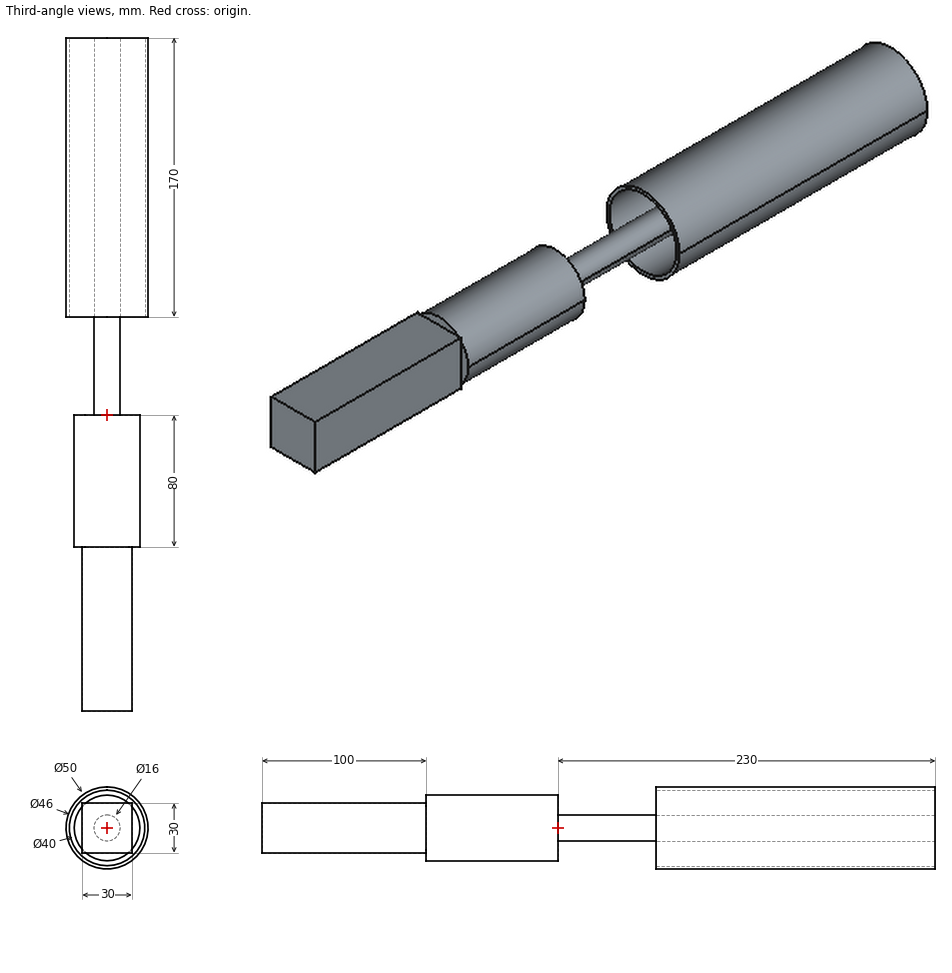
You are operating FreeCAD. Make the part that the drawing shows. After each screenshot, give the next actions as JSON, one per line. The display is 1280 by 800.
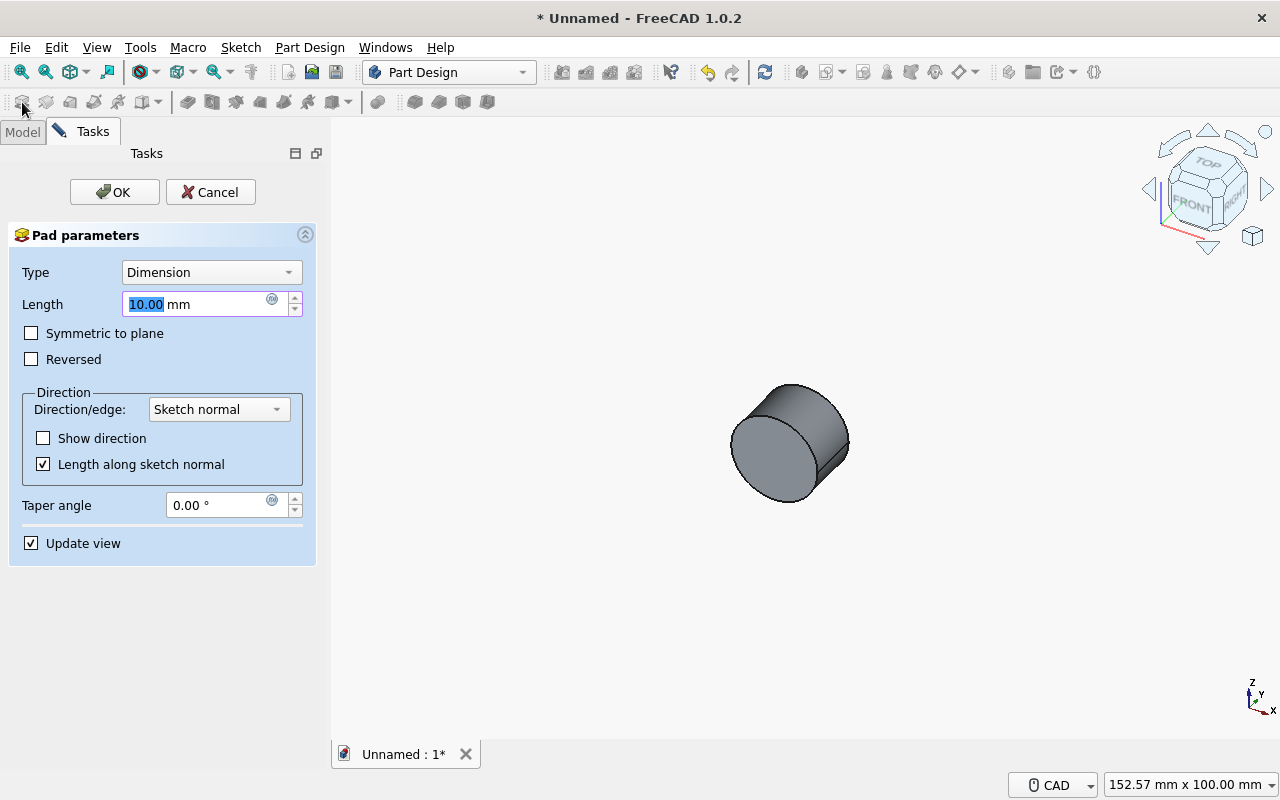
{"action": "type", "text": "230"}
{"action": "key", "text": "Tab"}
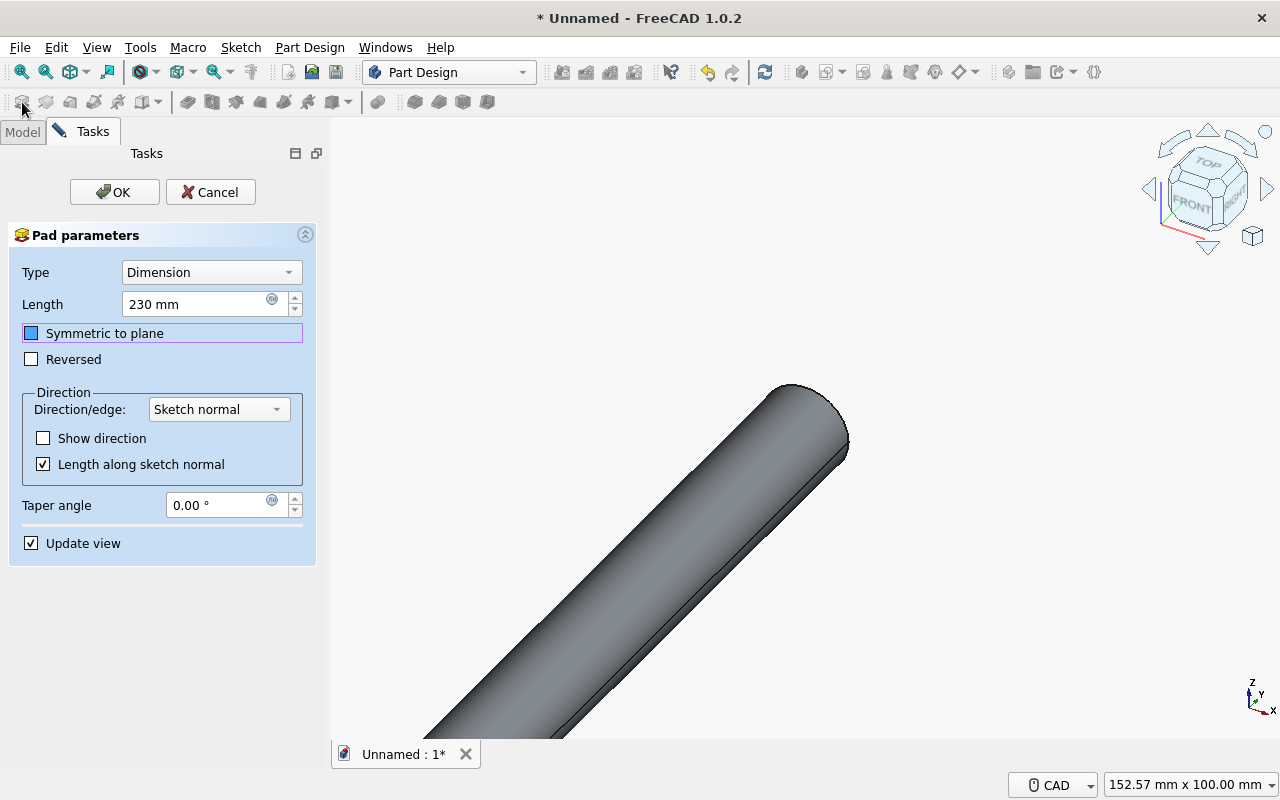
{"action": "left_click", "coordinate": [30, 359]}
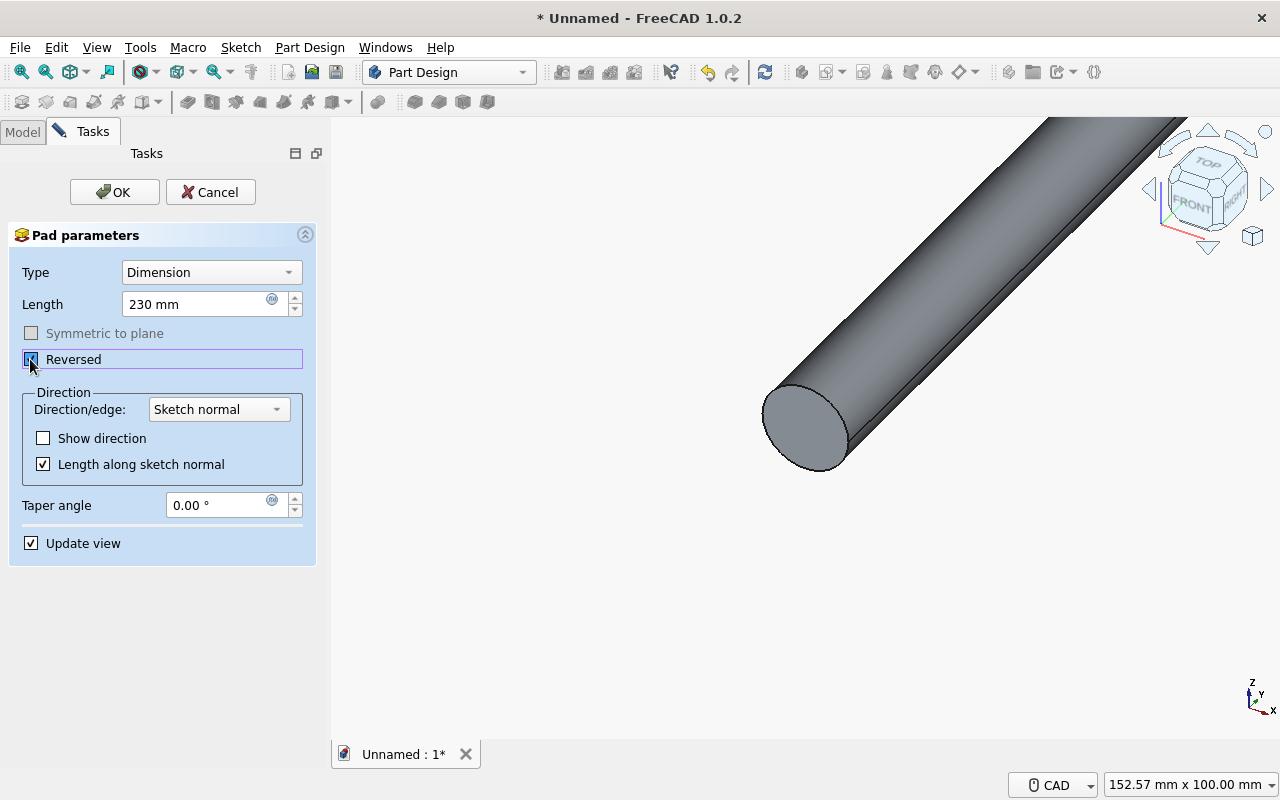
{"action": "left_click", "coordinate": [115, 192]}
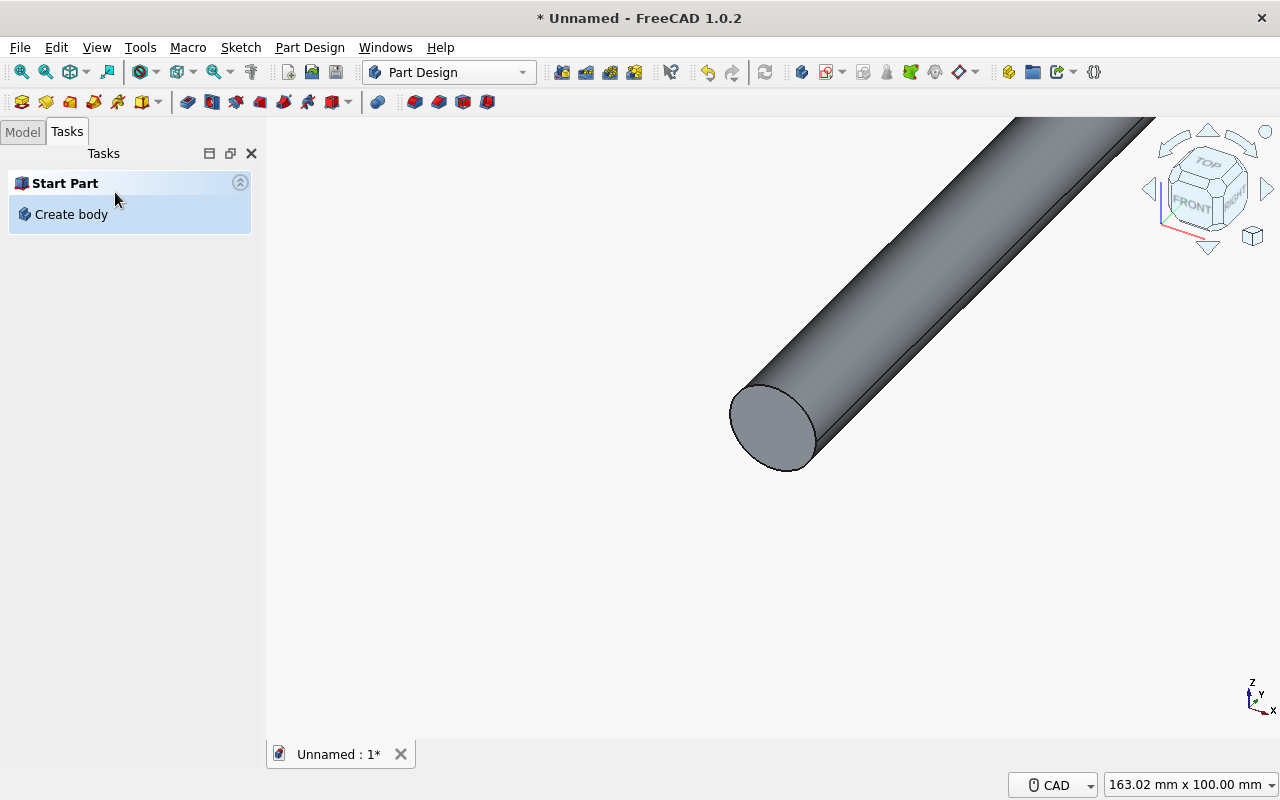
{"action": "left_click", "coordinate": [22, 72]}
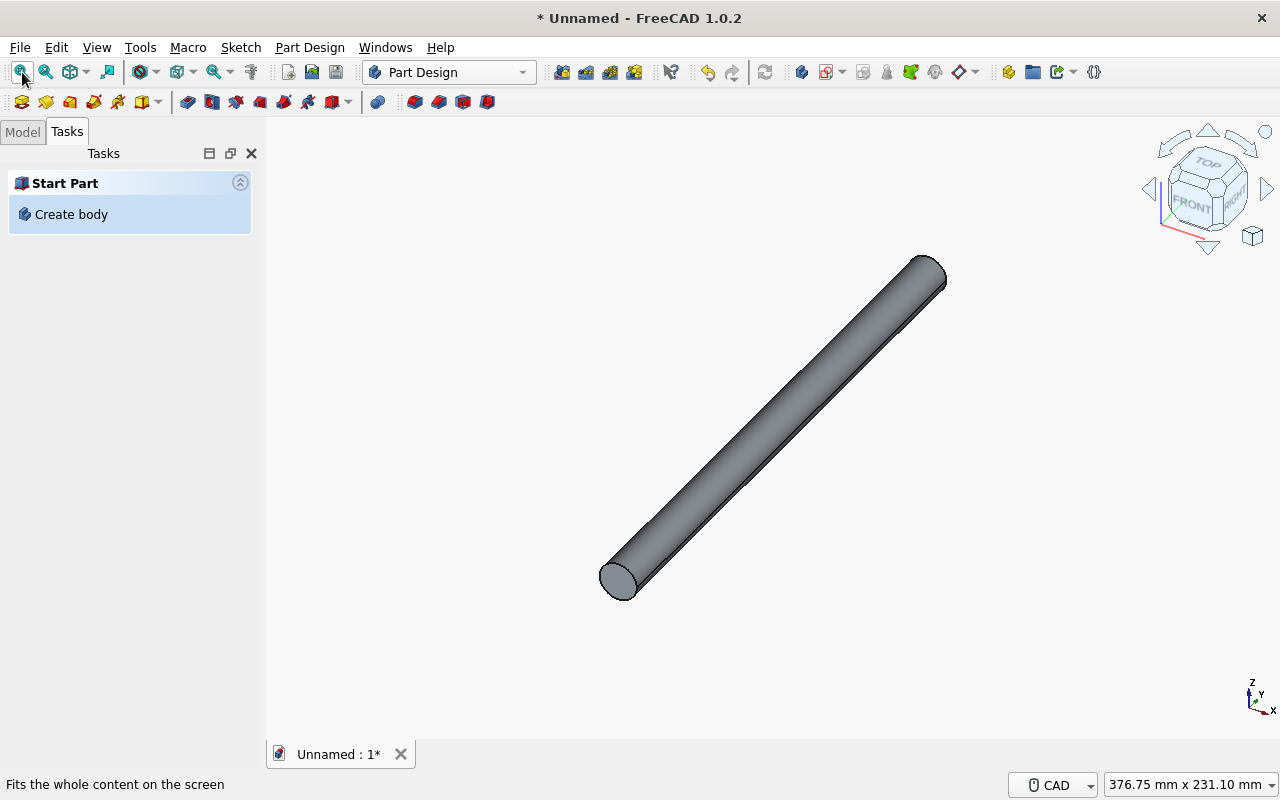
{"action": "left_click", "coordinate": [802, 72]}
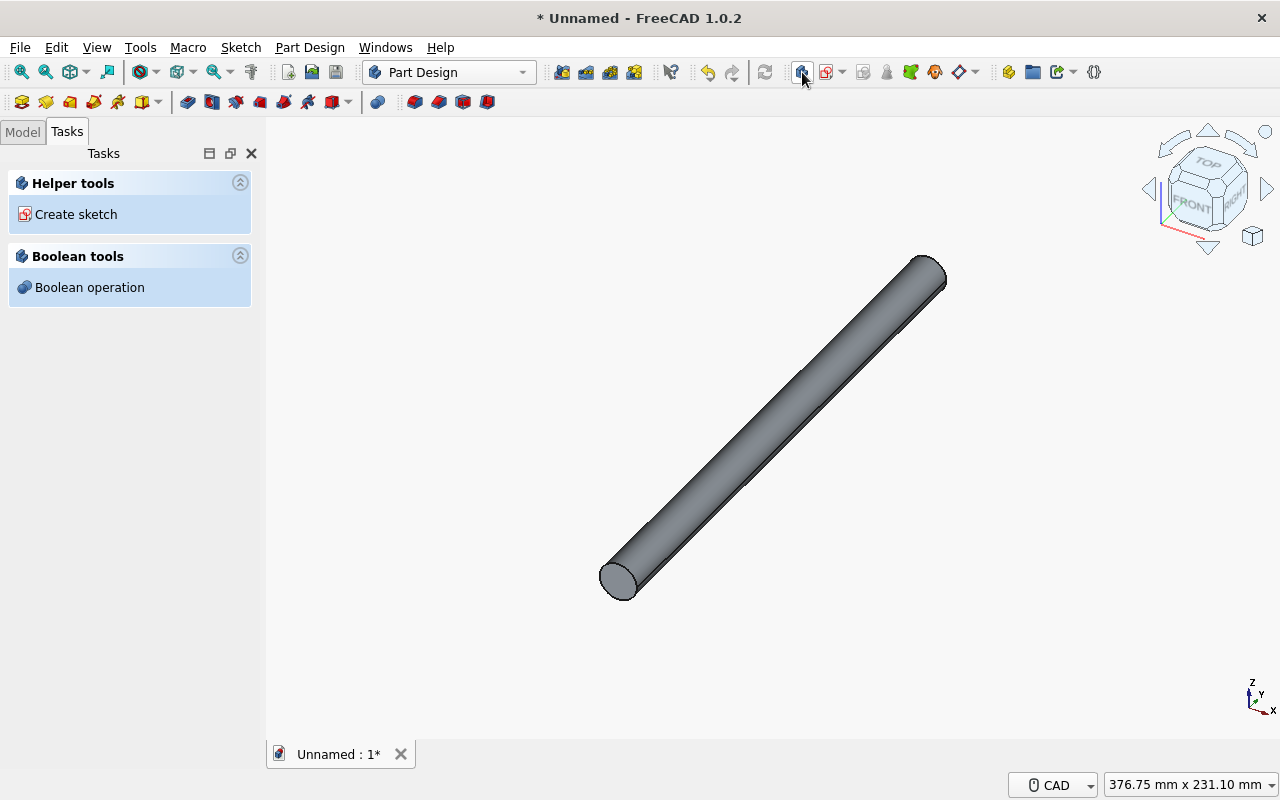
{"action": "left_click", "coordinate": [23, 131]}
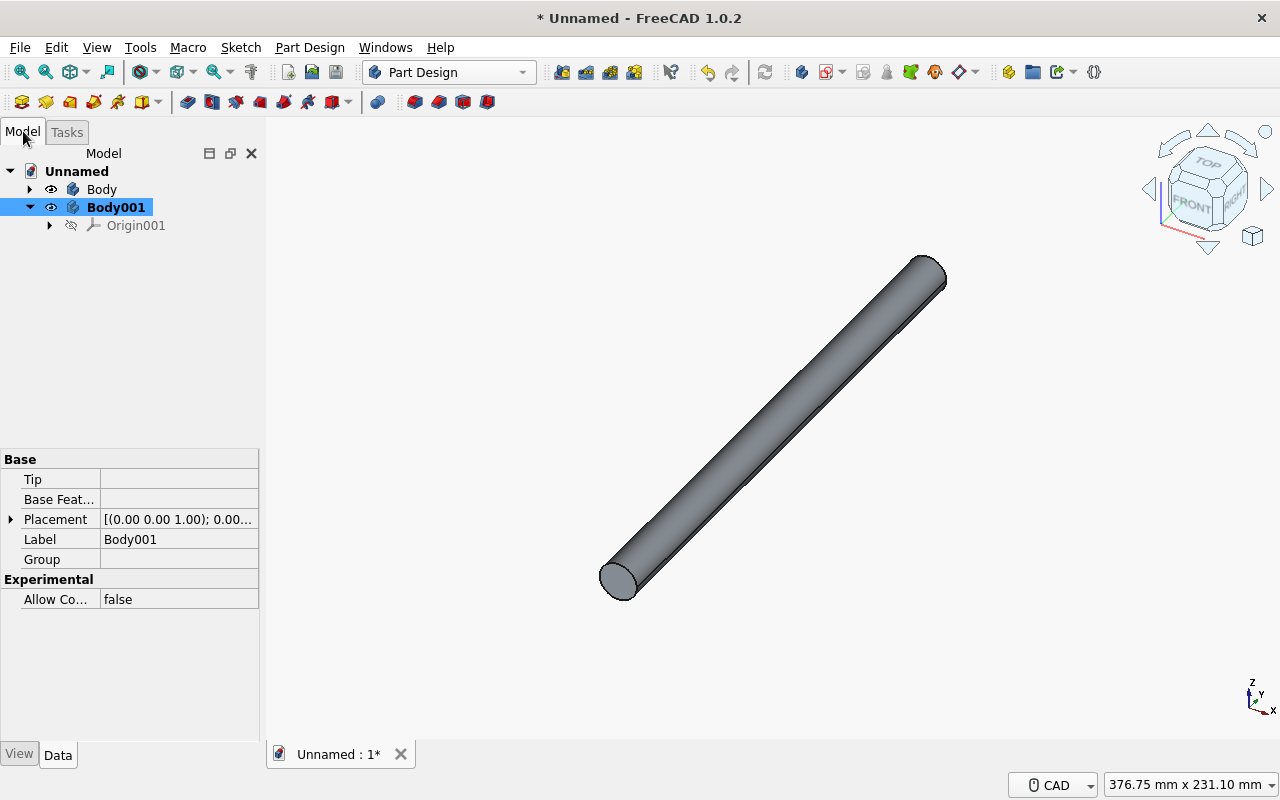
{"action": "left_click", "coordinate": [50, 225]}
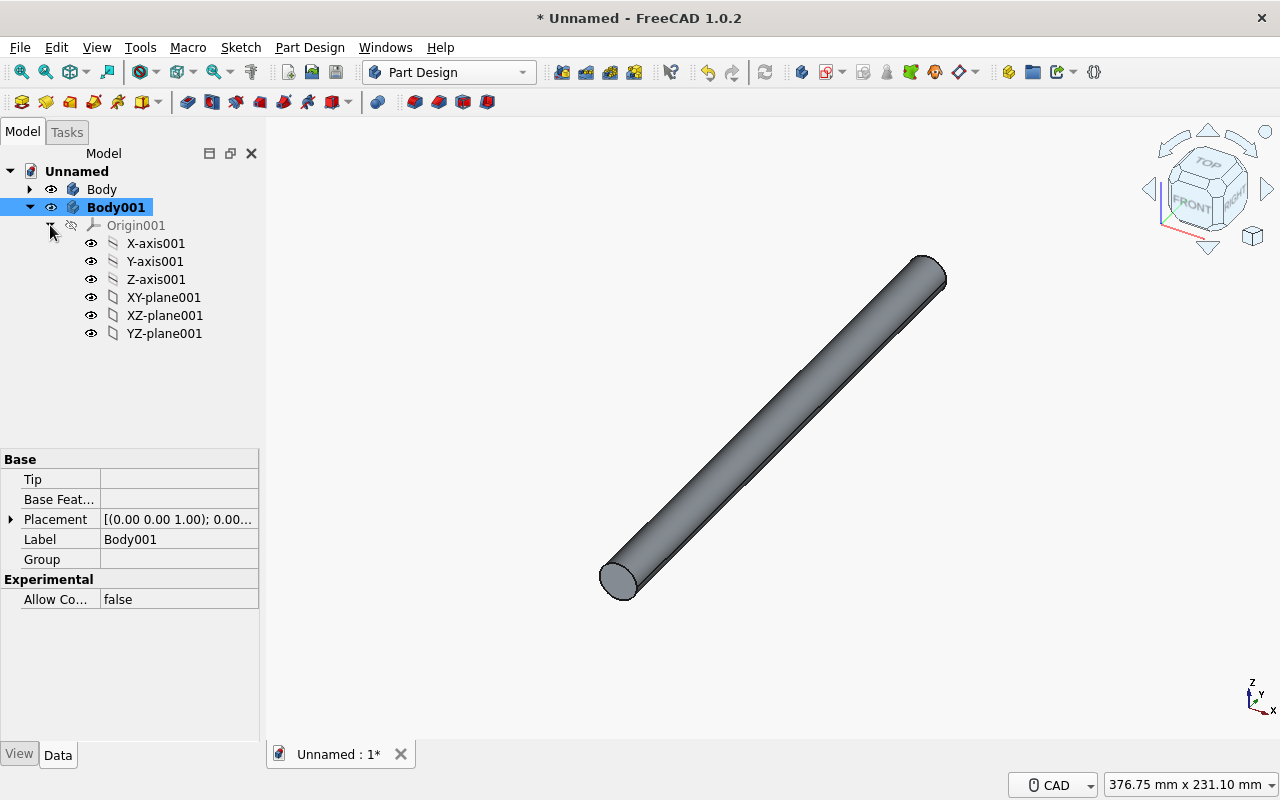
{"action": "left_click", "coordinate": [136, 315]}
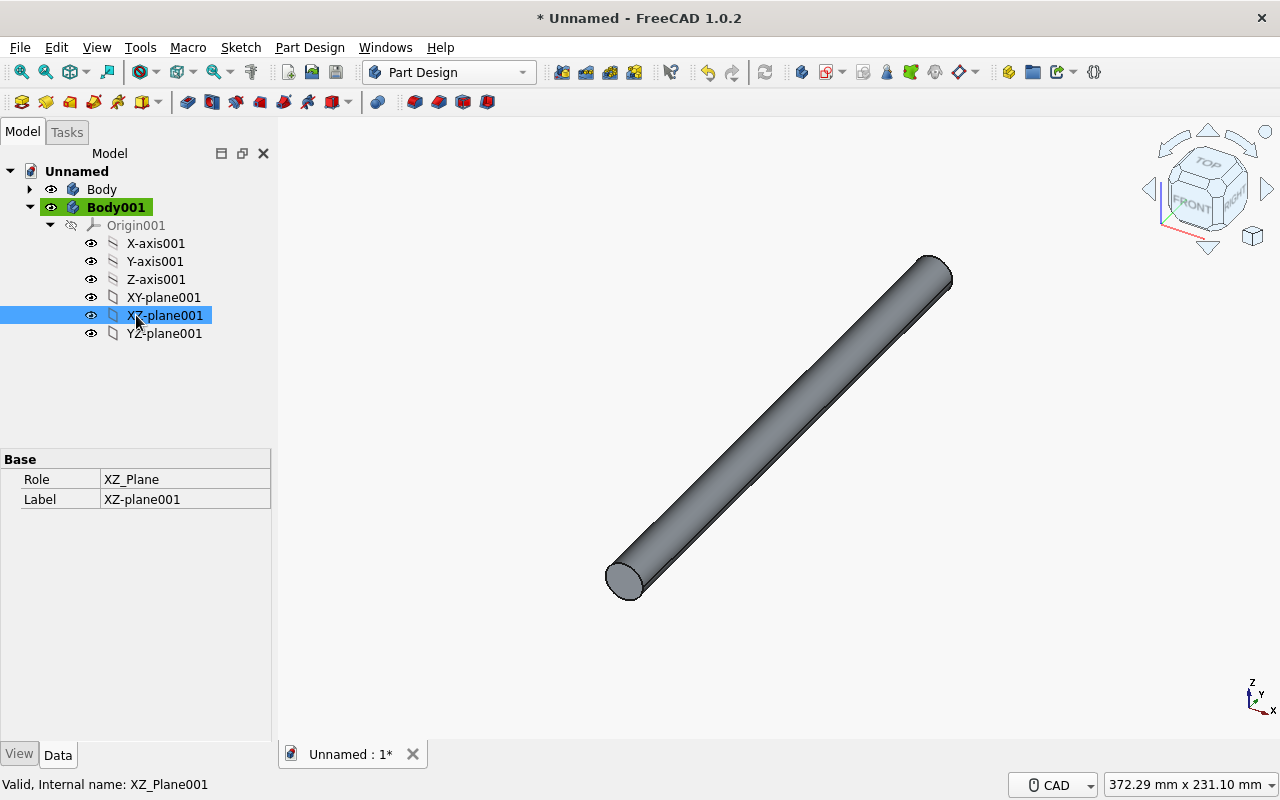
{"action": "left_click", "coordinate": [960, 72]}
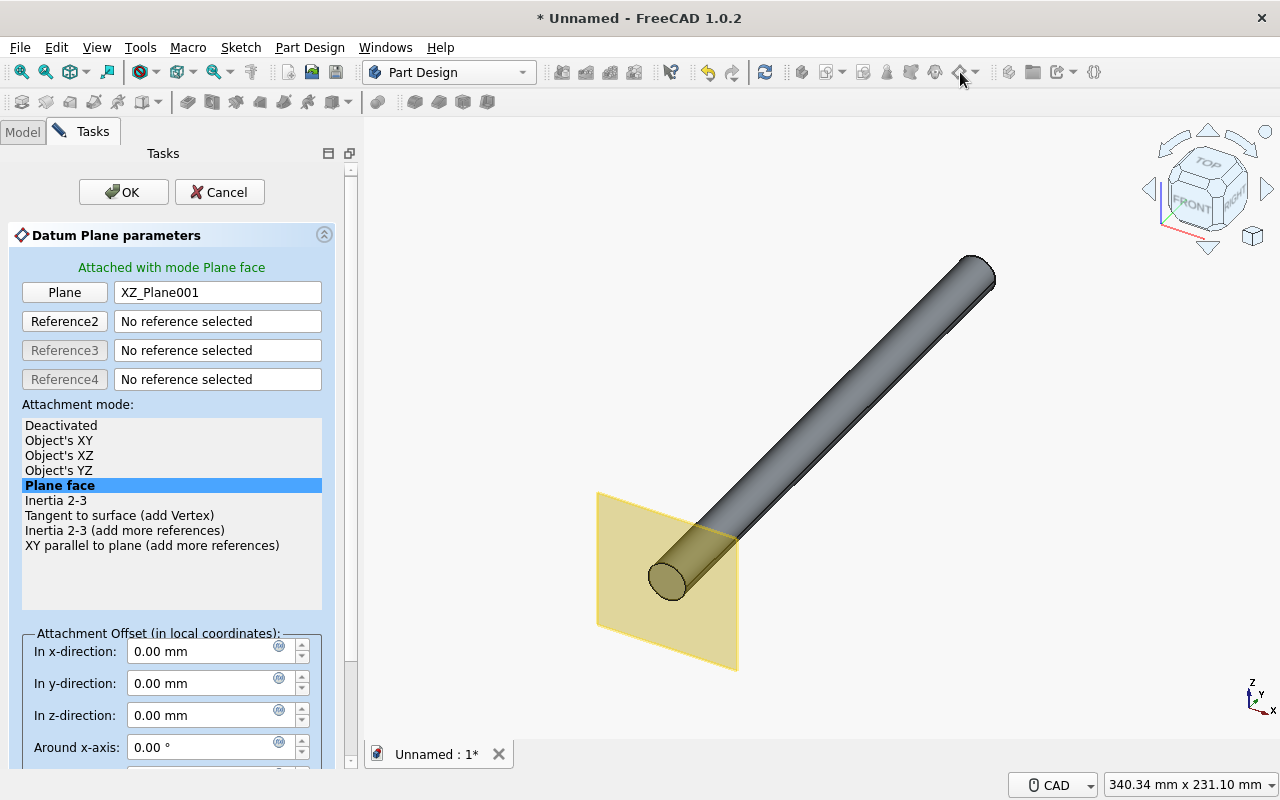
{"action": "triple_click", "coordinate": [210, 715]}